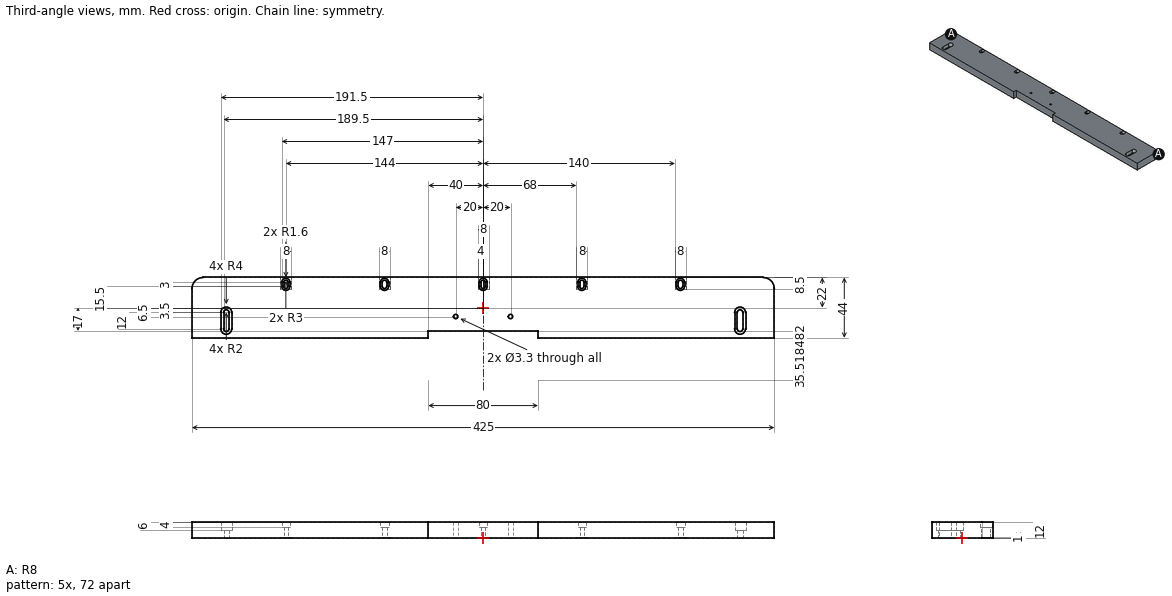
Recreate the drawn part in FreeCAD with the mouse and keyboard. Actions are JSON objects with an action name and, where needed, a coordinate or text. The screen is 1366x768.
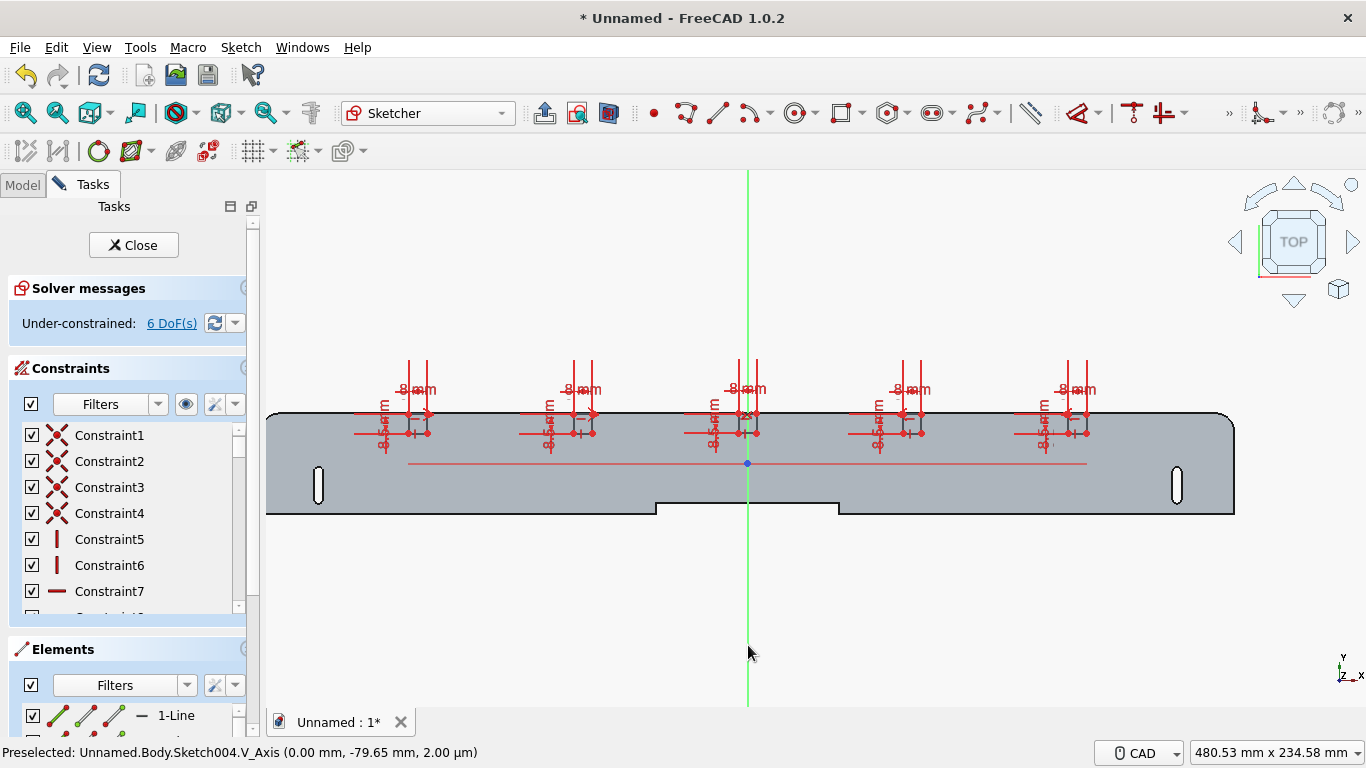
{"action": "key", "text": "d"}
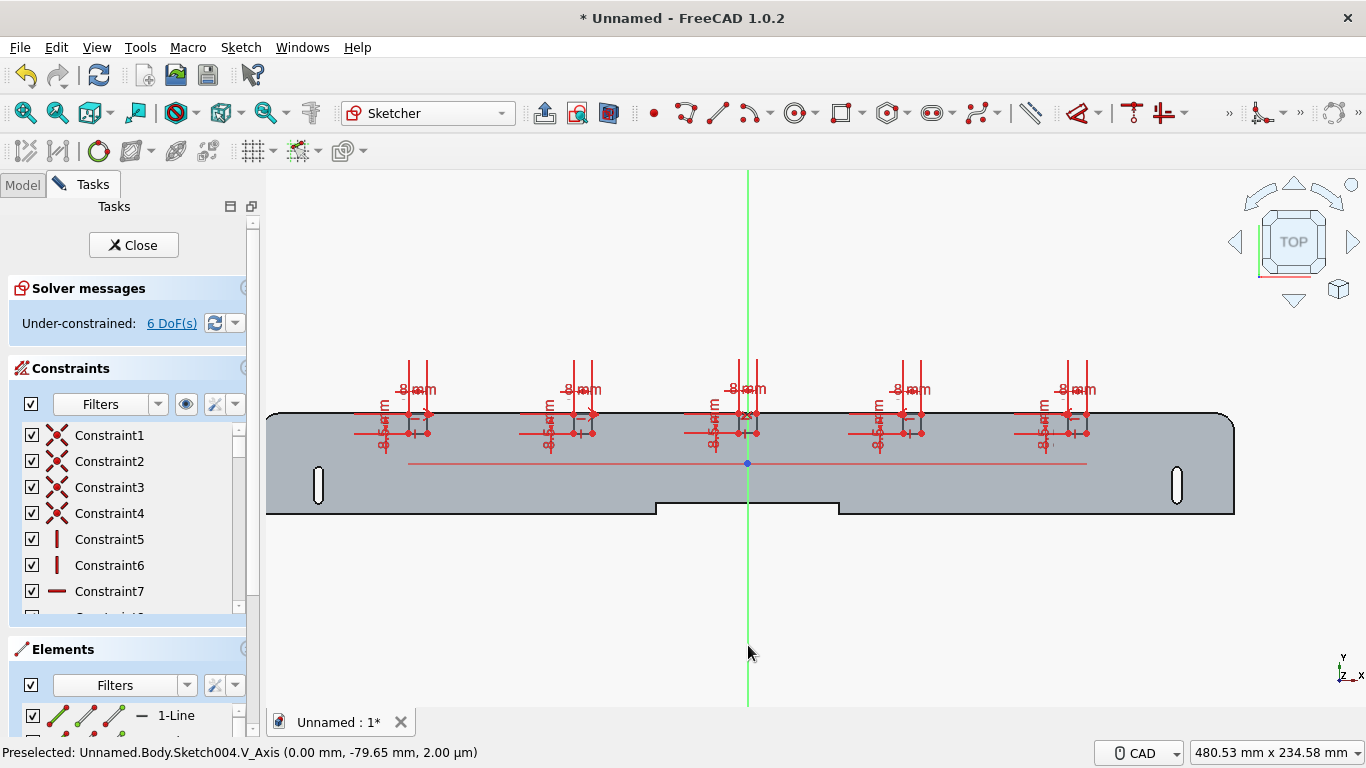
{"action": "scroll", "coordinate": [739, 414], "scroll_direction": "up", "scroll_amount": 8}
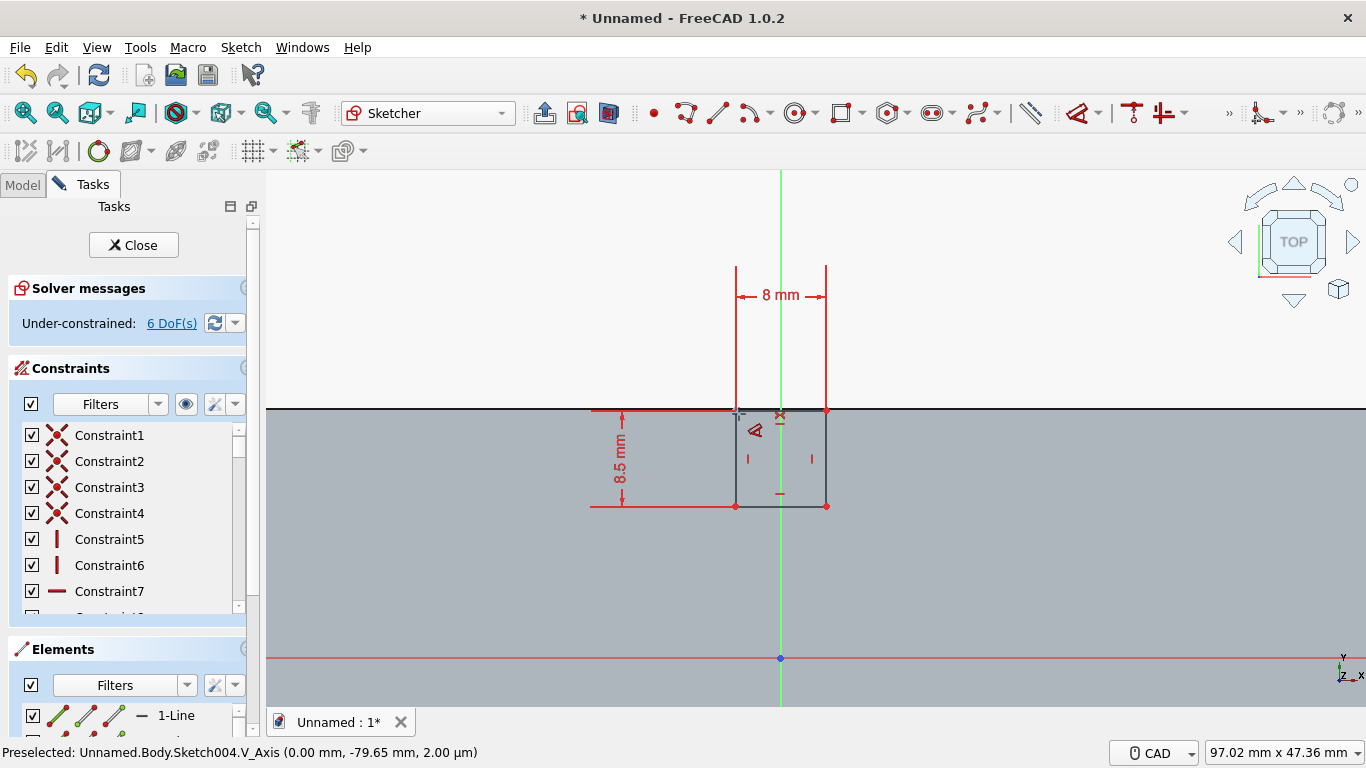
{"action": "left_click", "coordinate": [736, 410]}
{"action": "left_click", "coordinate": [758, 376]}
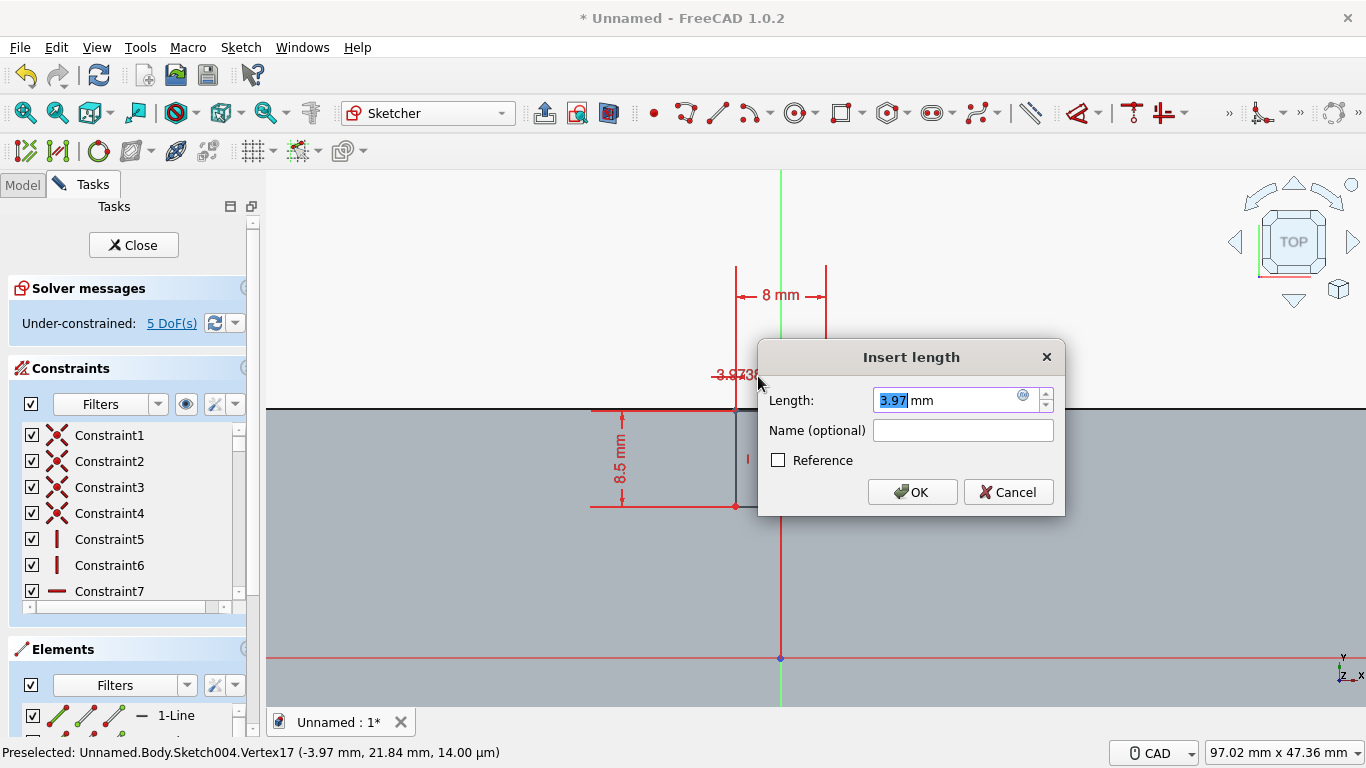
{"action": "type", "text": "4"}
{"action": "key", "text": "Return"}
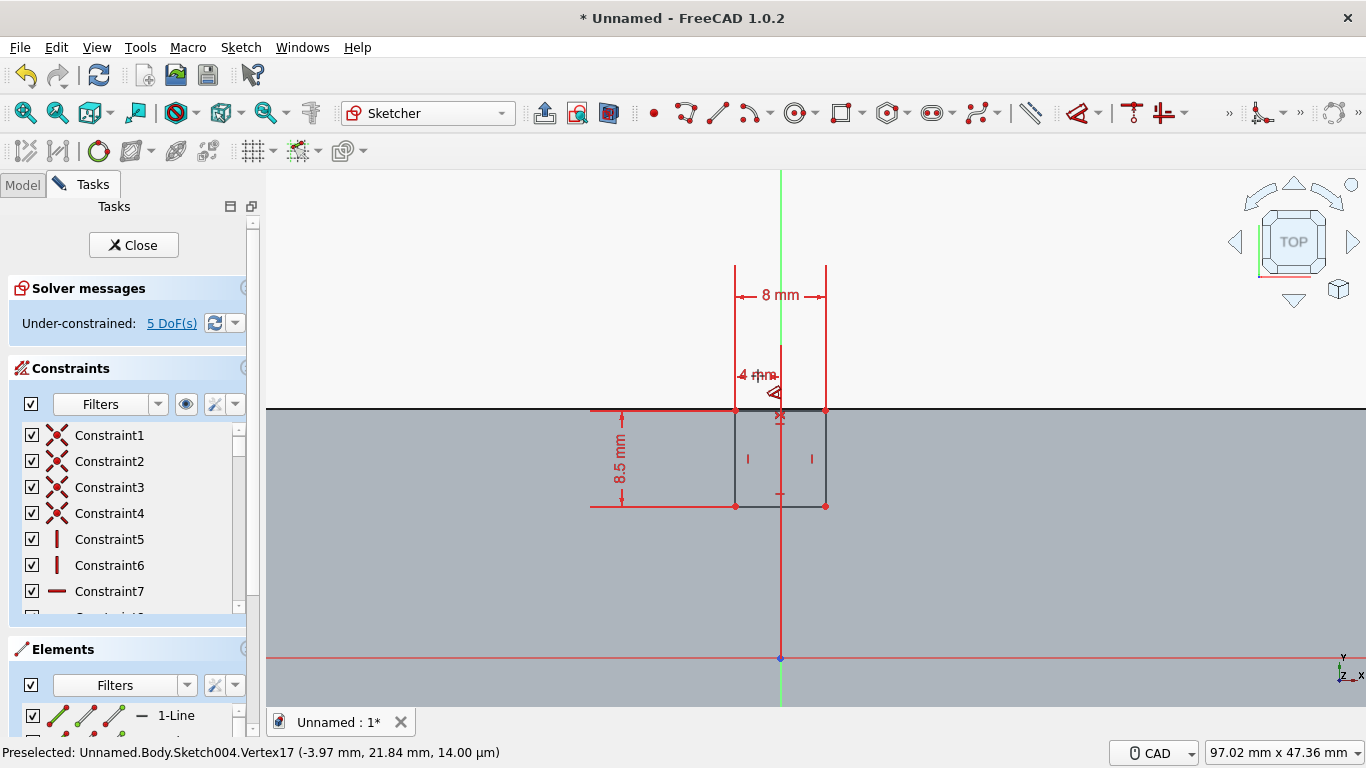
{"action": "scroll", "coordinate": [739, 414], "scroll_direction": "down", "scroll_amount": 8}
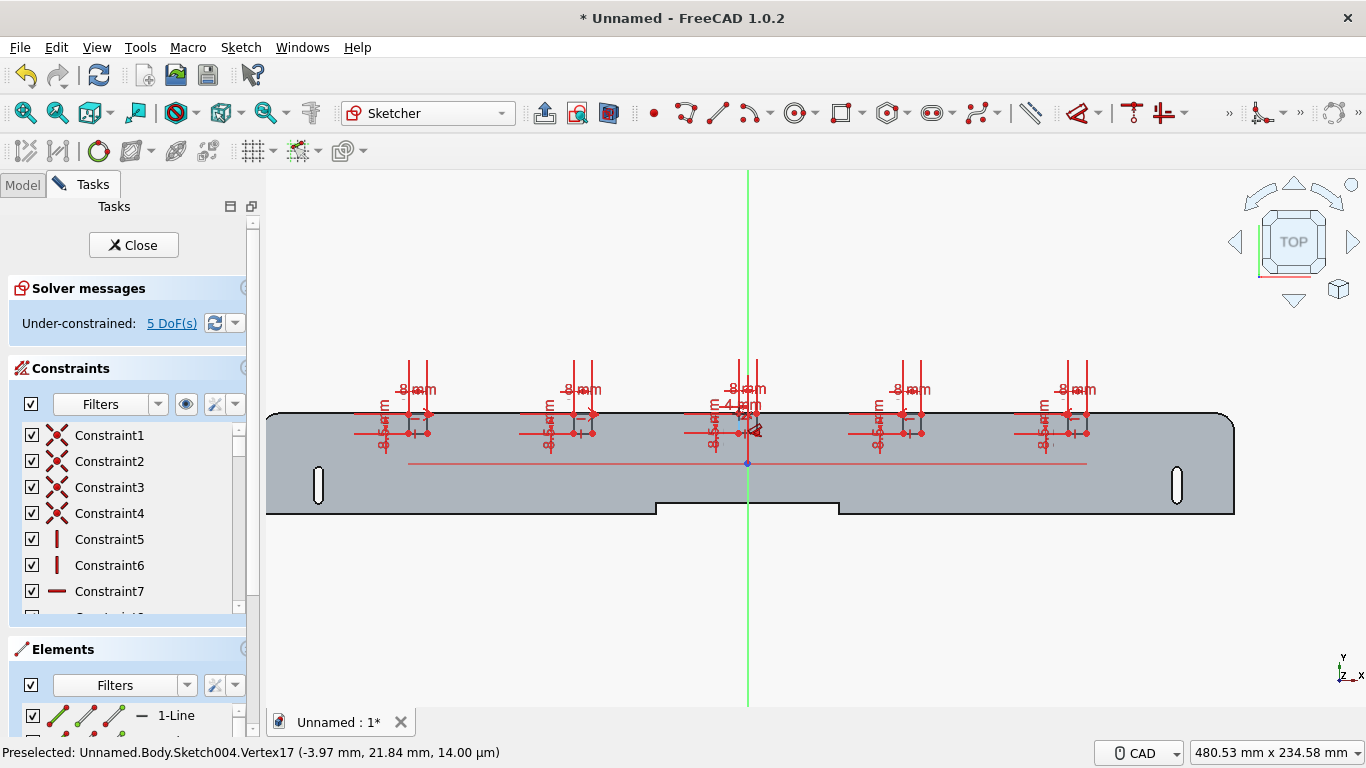
{"action": "left_click", "coordinate": [1068, 414]}
{"action": "left_click", "coordinate": [1102, 439]}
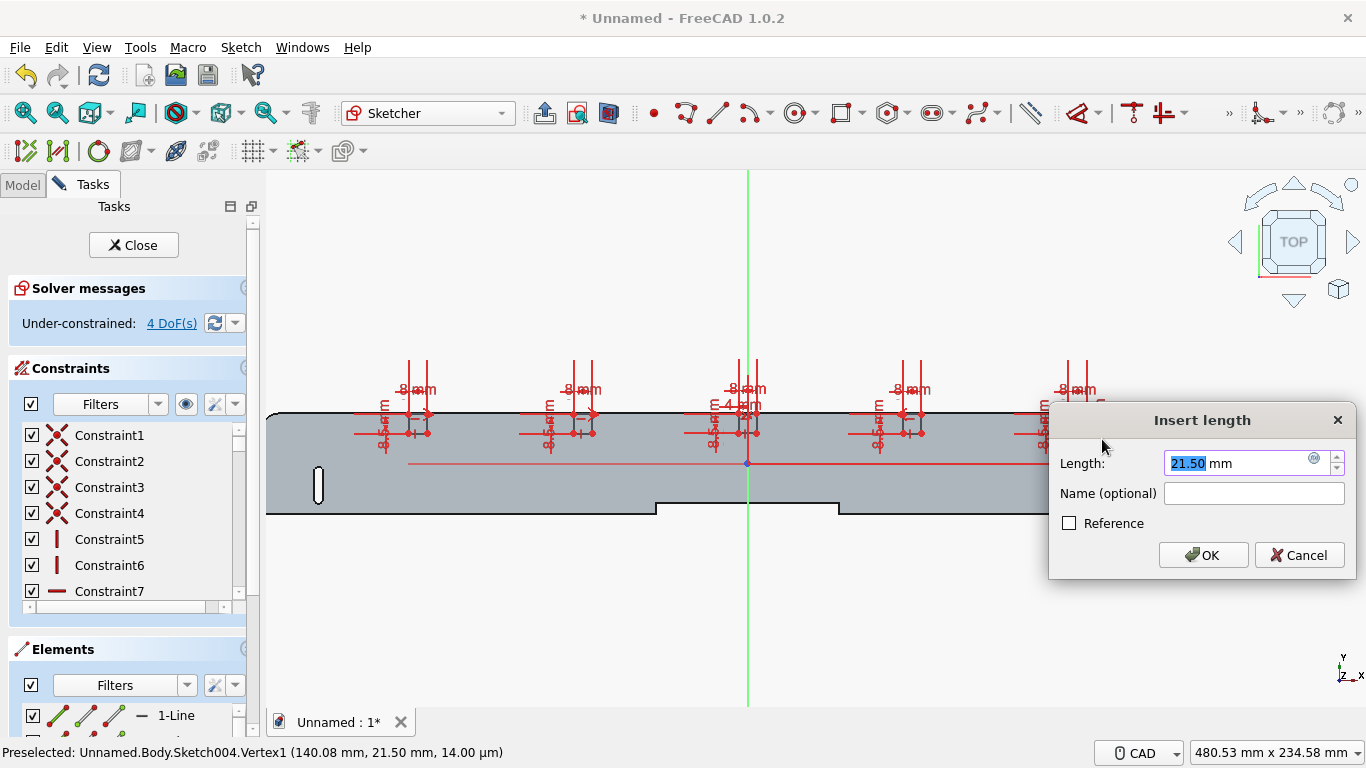
{"action": "type", "text": "22"}
{"action": "key", "text": "Return"}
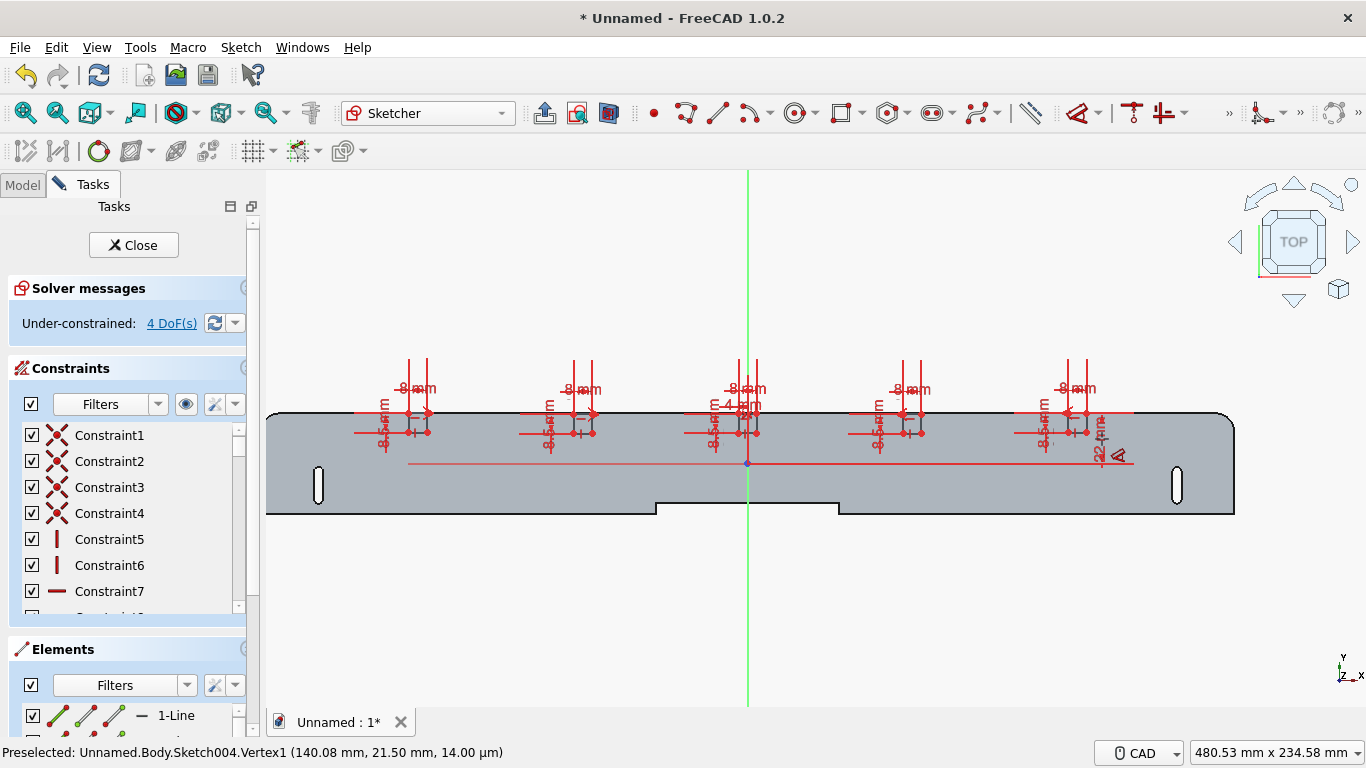
{"action": "left_click", "coordinate": [903, 414]}
{"action": "left_click", "coordinate": [825, 498]}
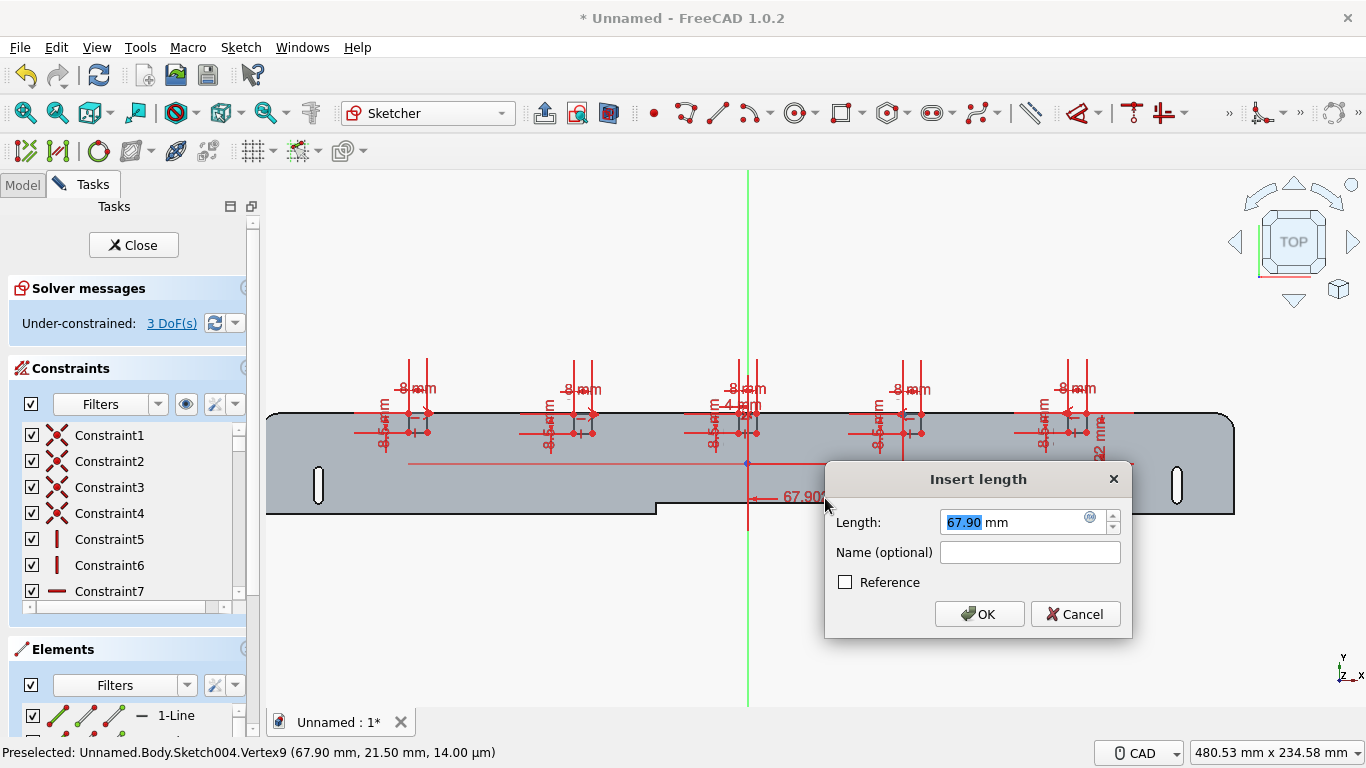
{"action": "type", "text": "68"}
{"action": "key", "text": "Return"}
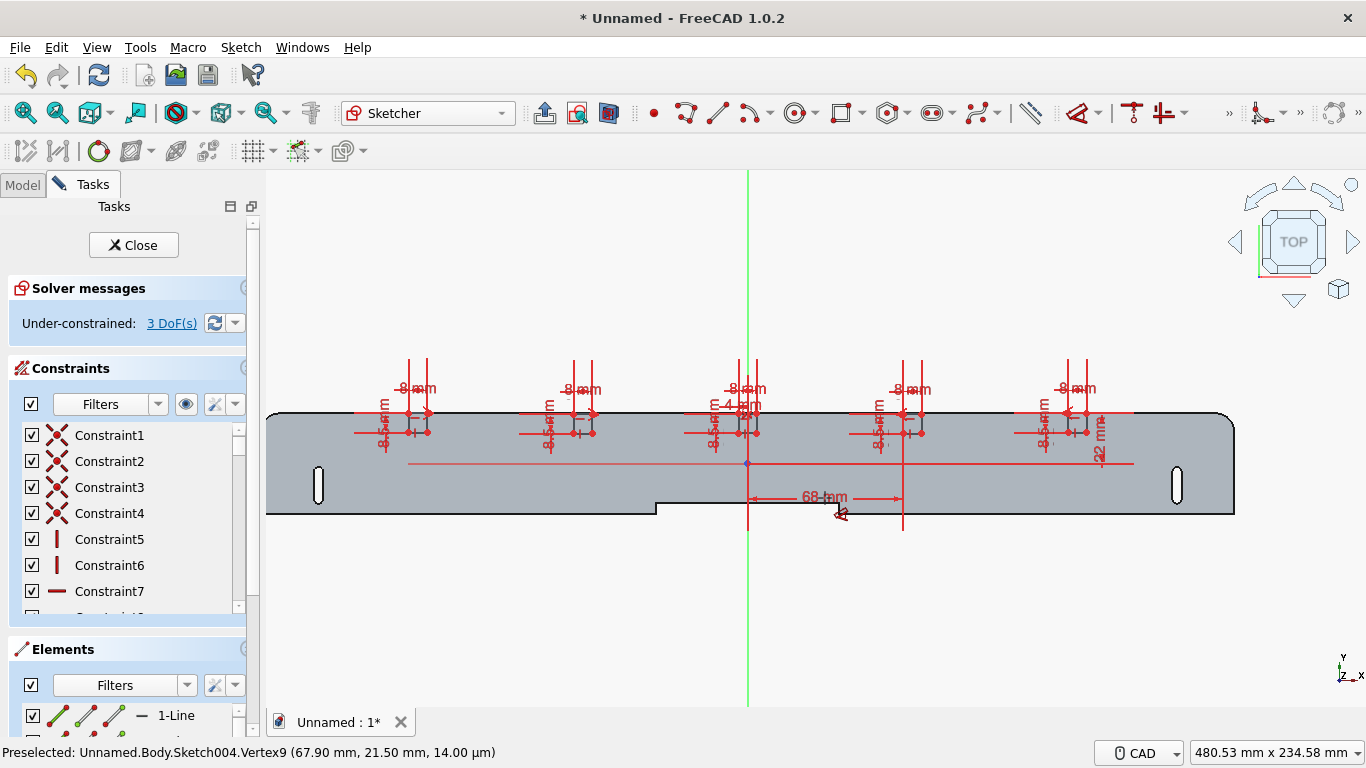
{"action": "left_click", "coordinate": [903, 414]}
{"action": "left_click", "coordinate": [937, 439]}